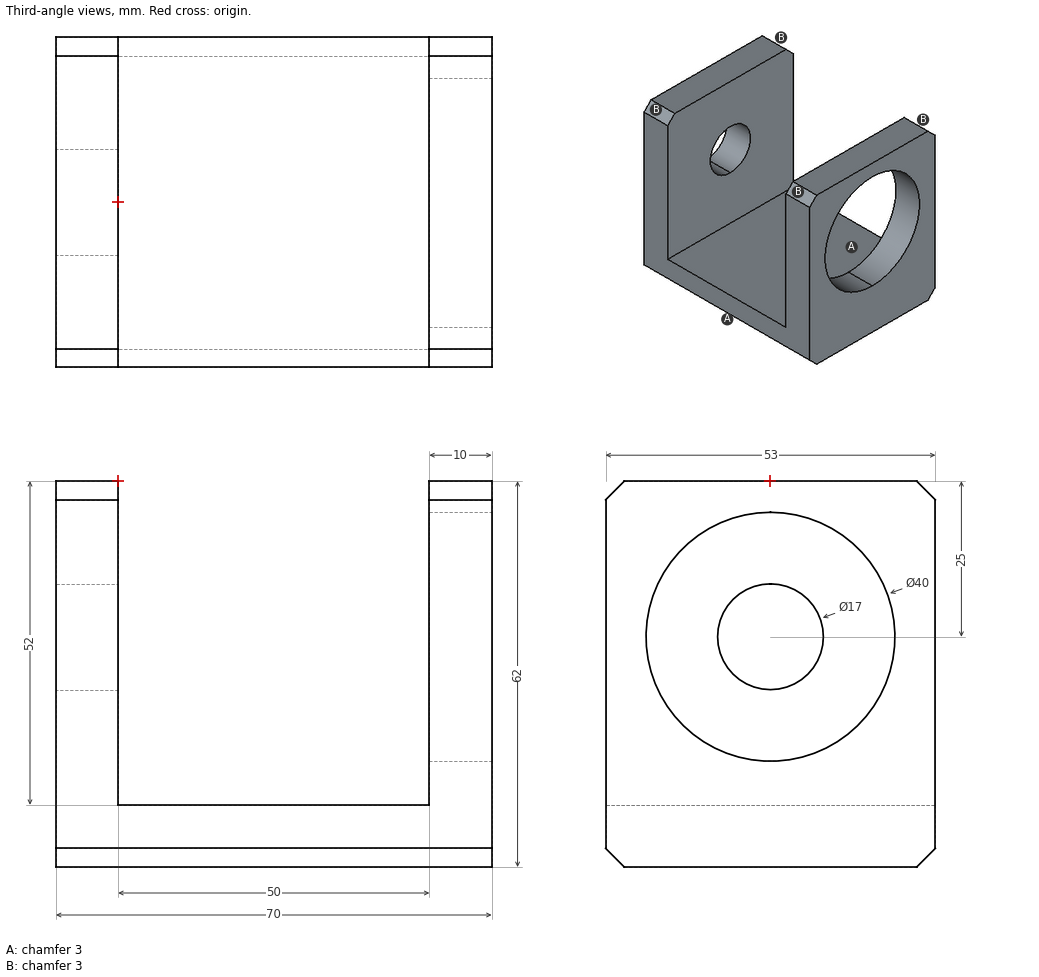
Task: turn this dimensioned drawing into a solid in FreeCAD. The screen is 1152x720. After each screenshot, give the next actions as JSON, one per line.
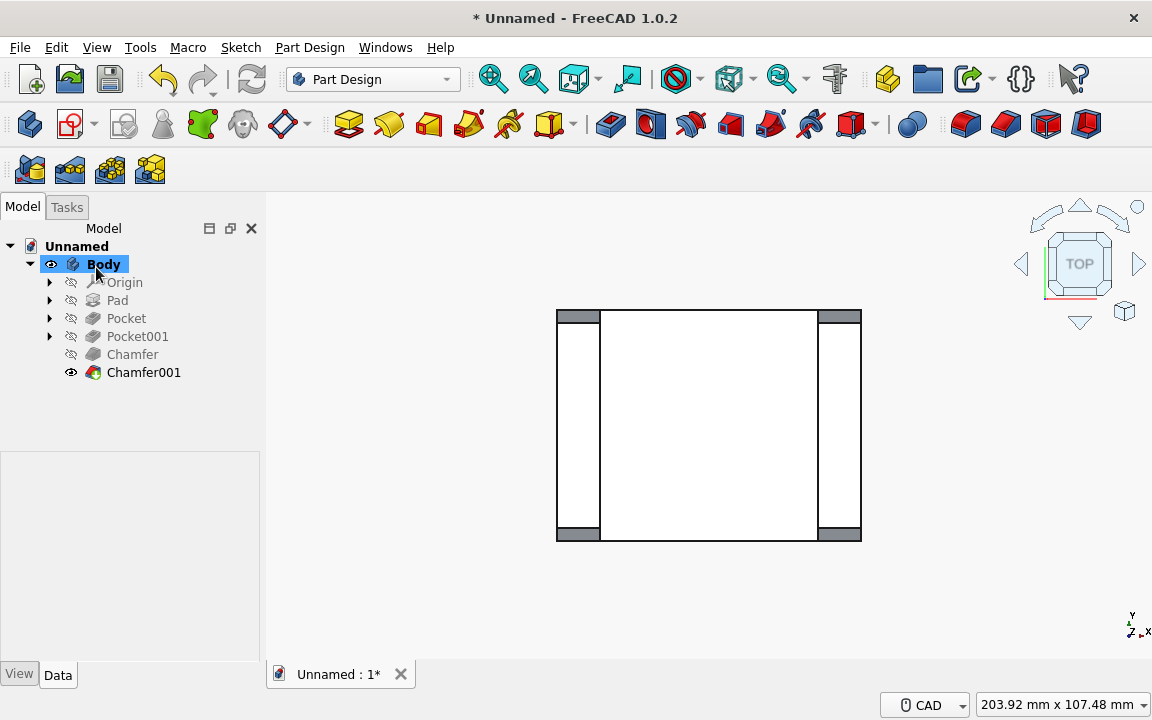
{"action": "key", "text": "0"}